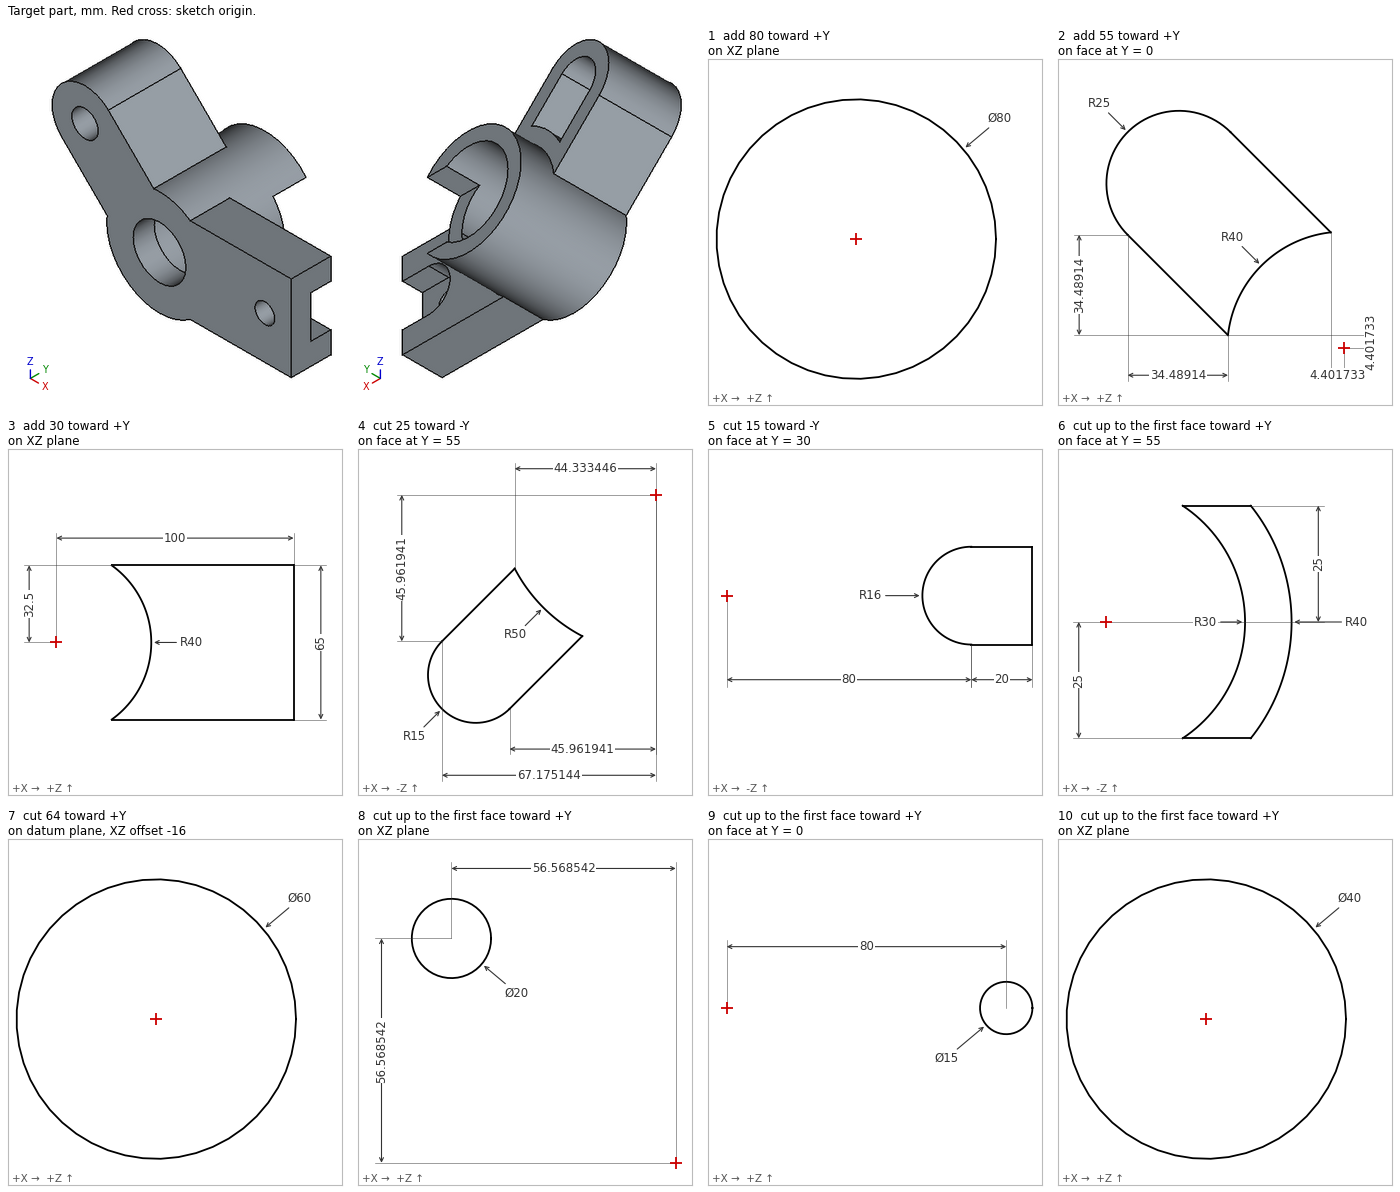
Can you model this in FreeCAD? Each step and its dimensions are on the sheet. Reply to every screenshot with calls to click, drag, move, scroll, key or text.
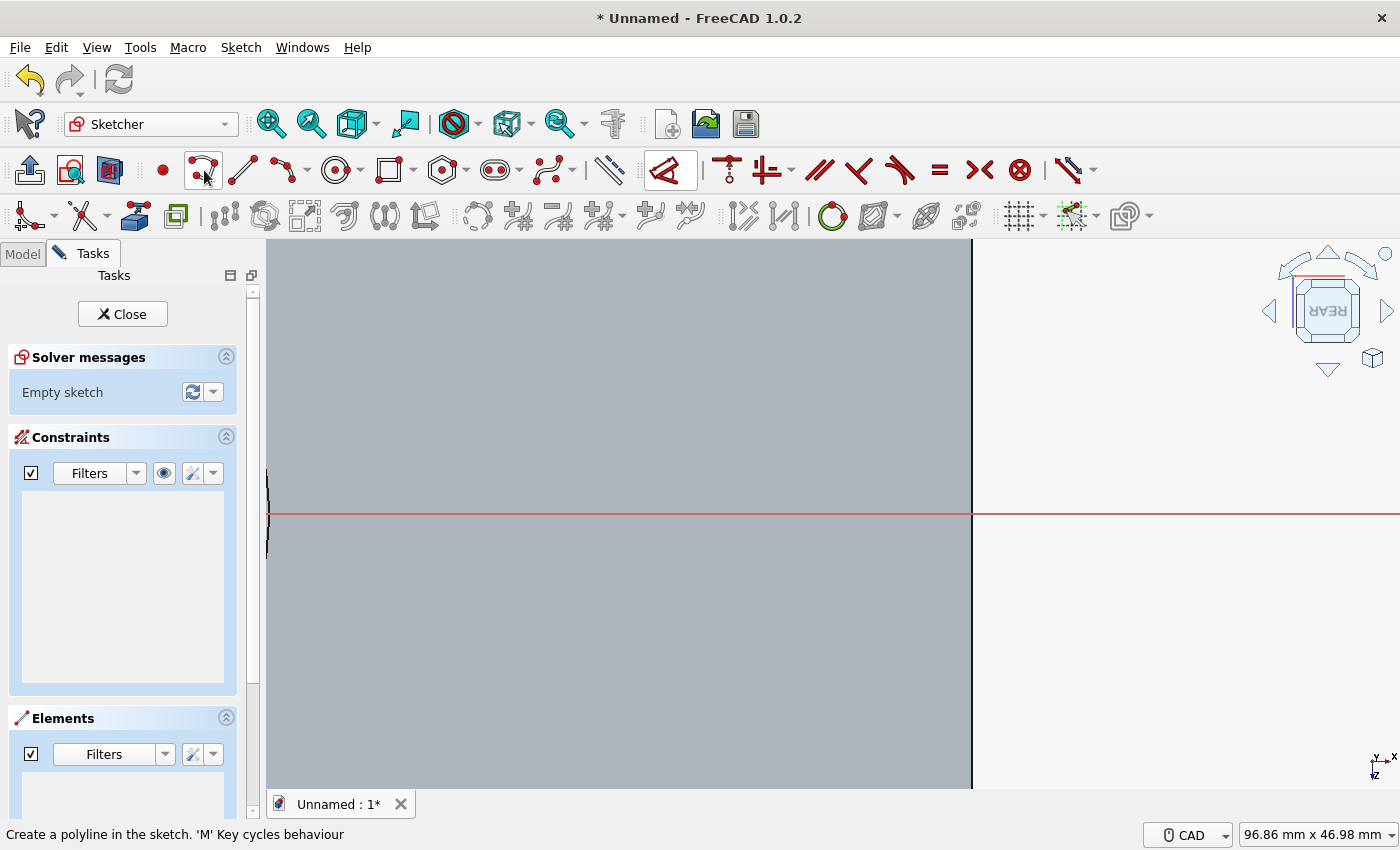
click(738, 702)
click(972, 702)
click(972, 327)
click(738, 327)
right_click(738, 327)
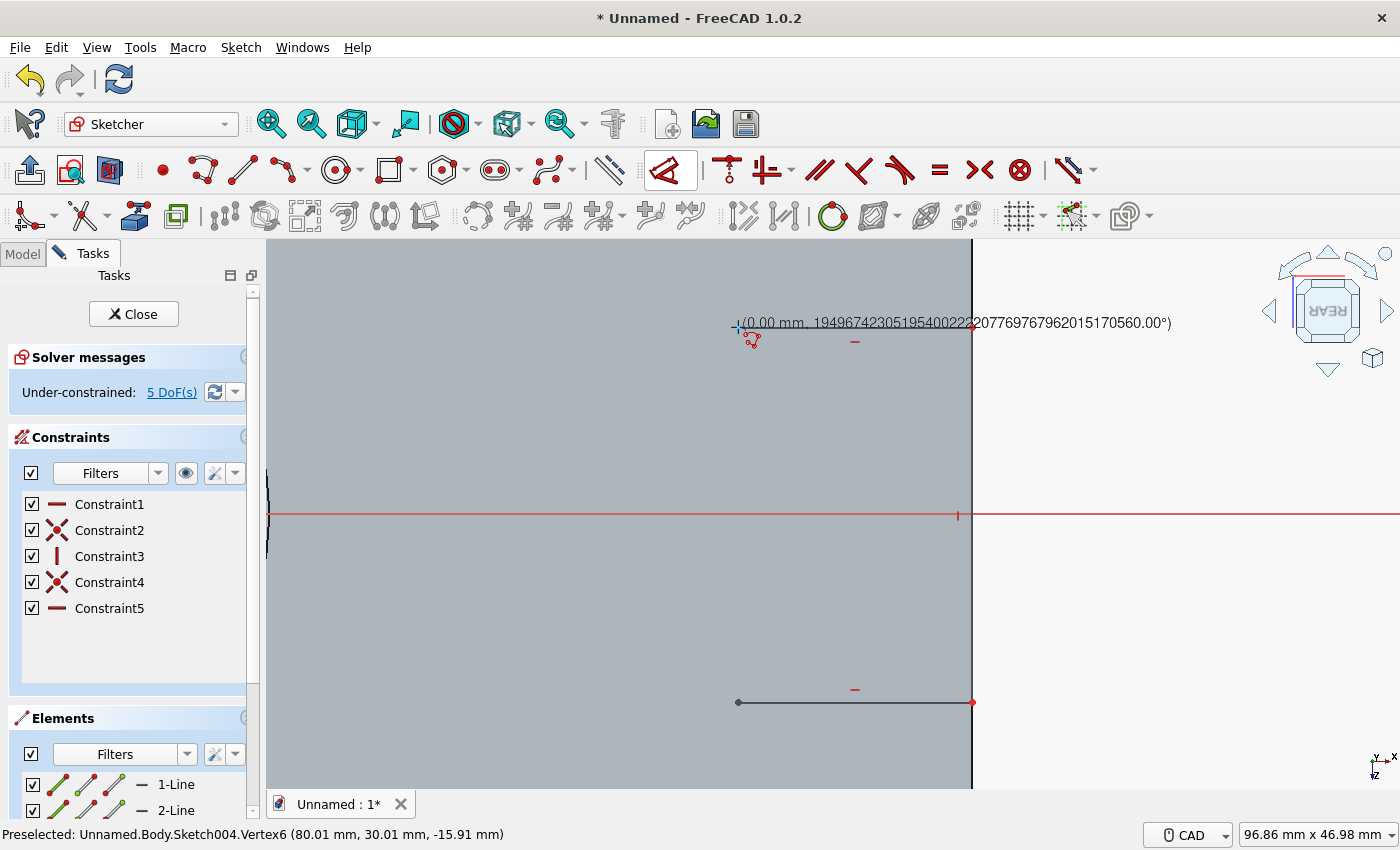
click(284, 170)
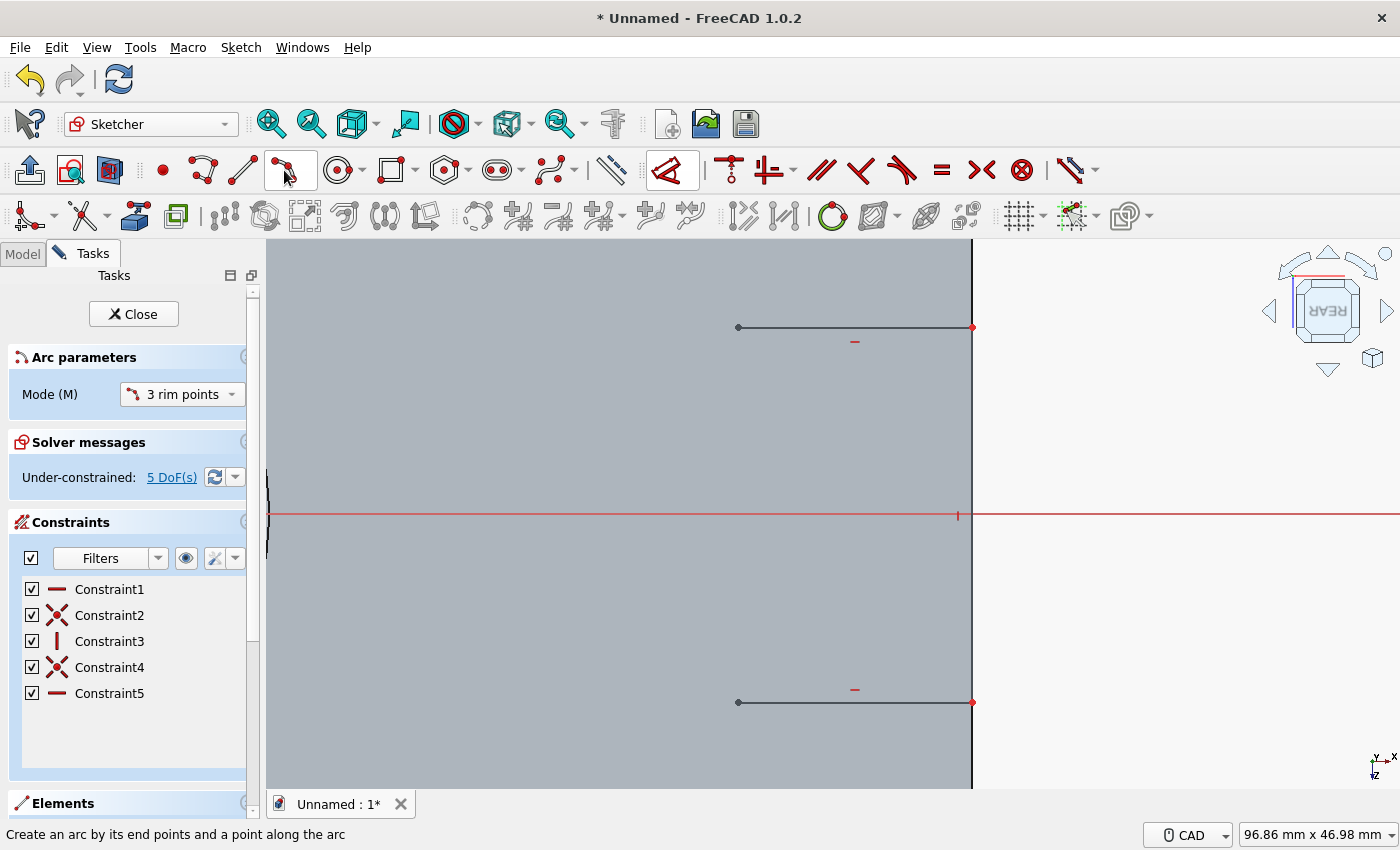
click(738, 328)
click(738, 703)
click(560, 456)
key(Escape)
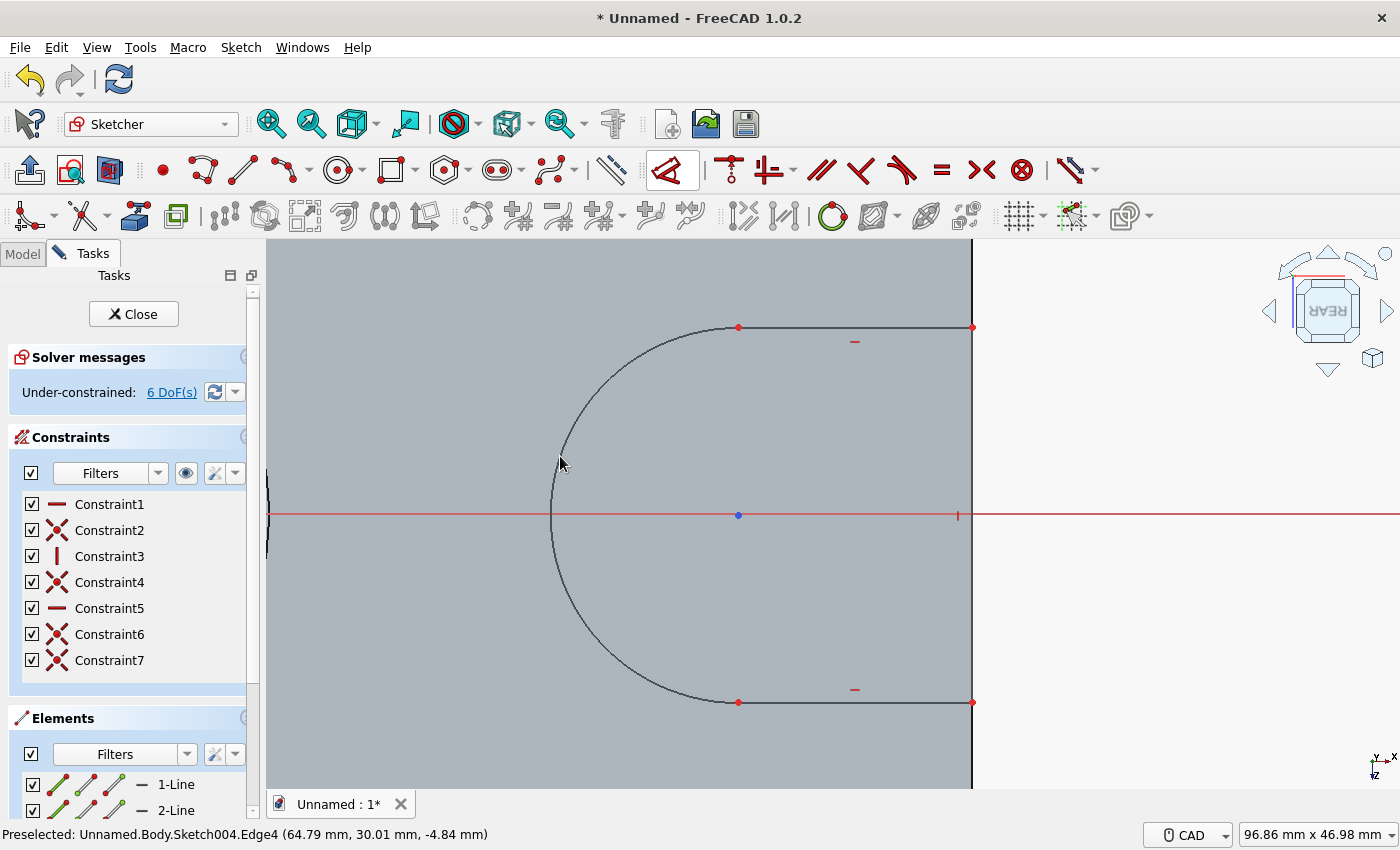
click(808, 703)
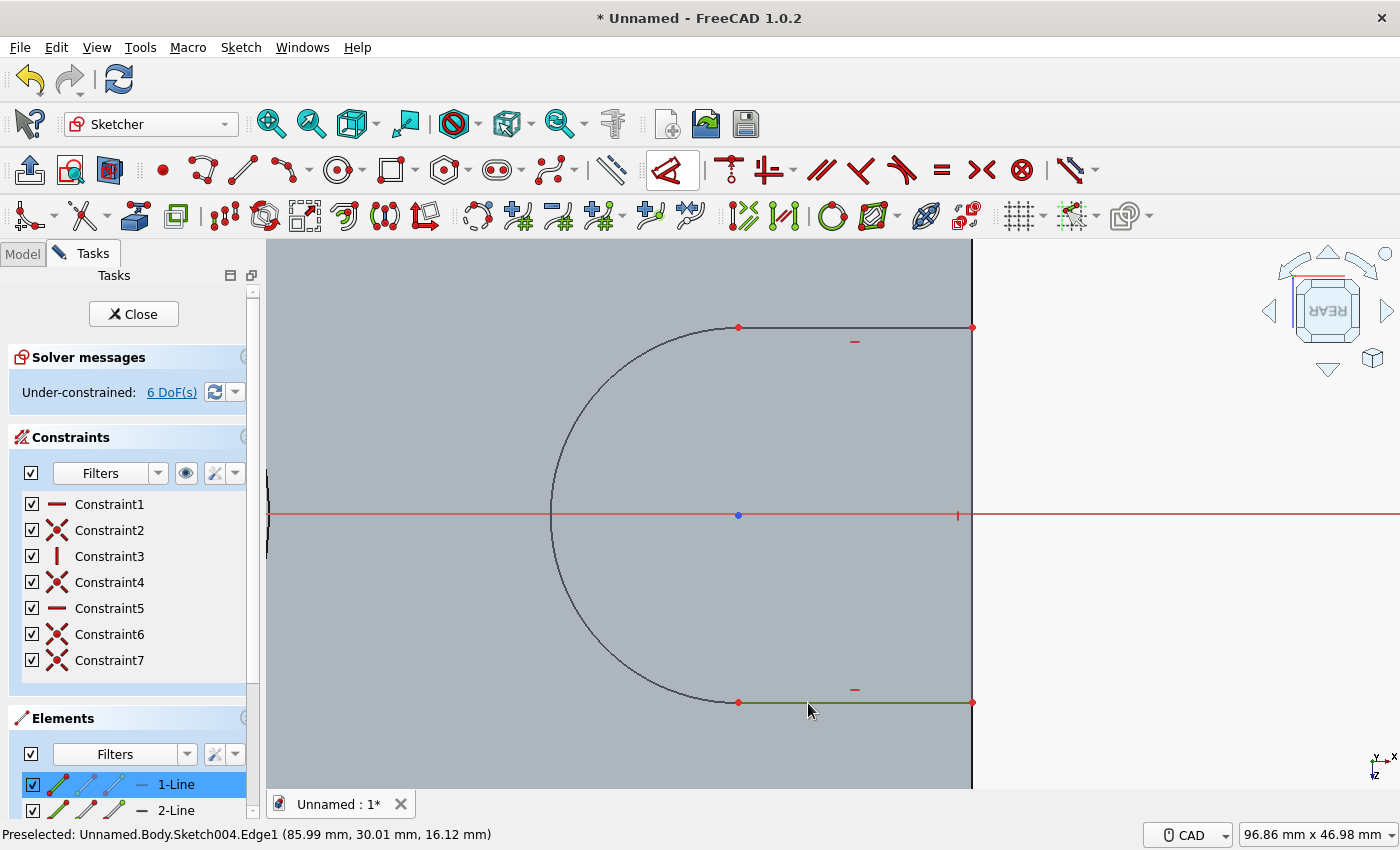
click(586, 405)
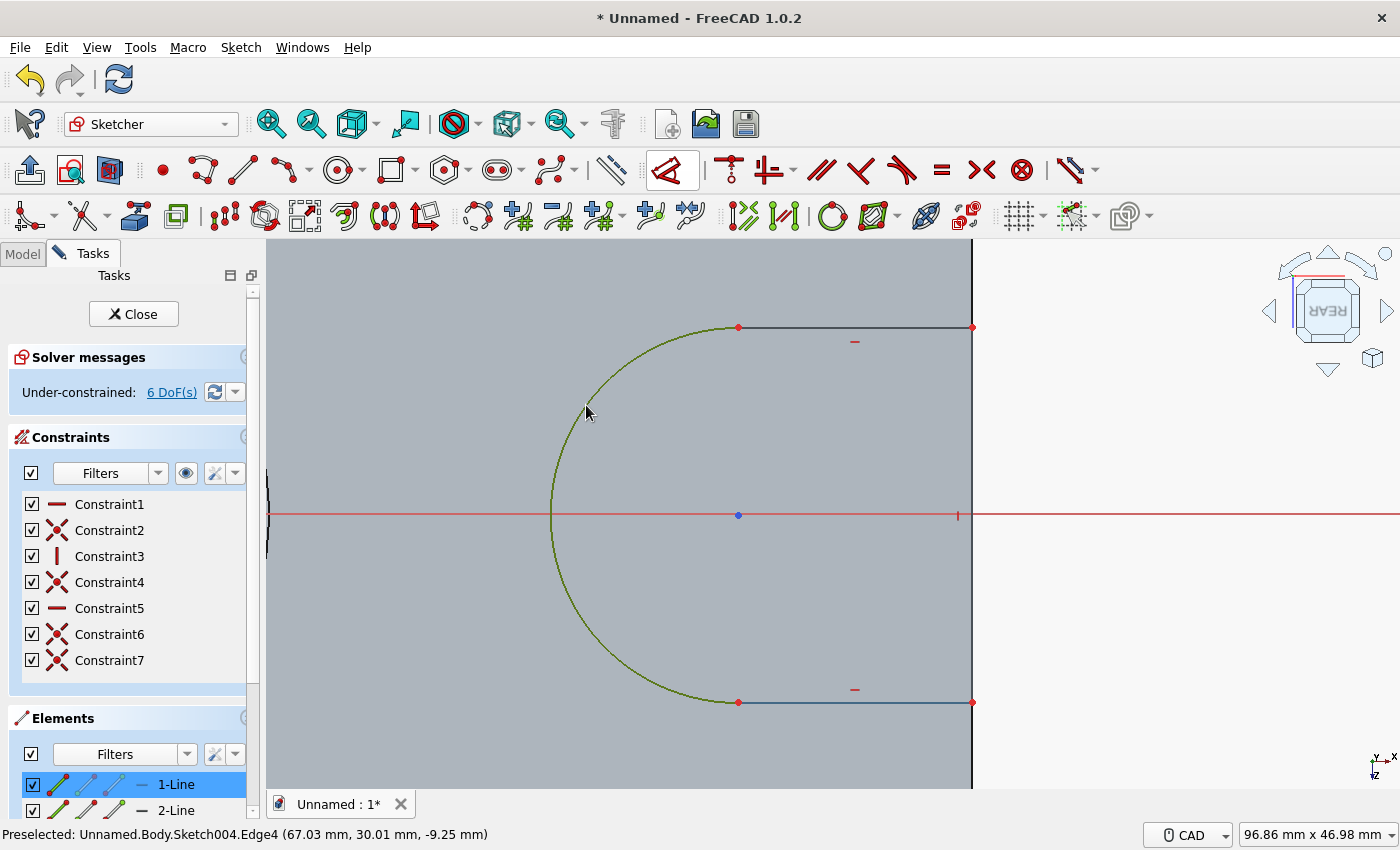
click(902, 170)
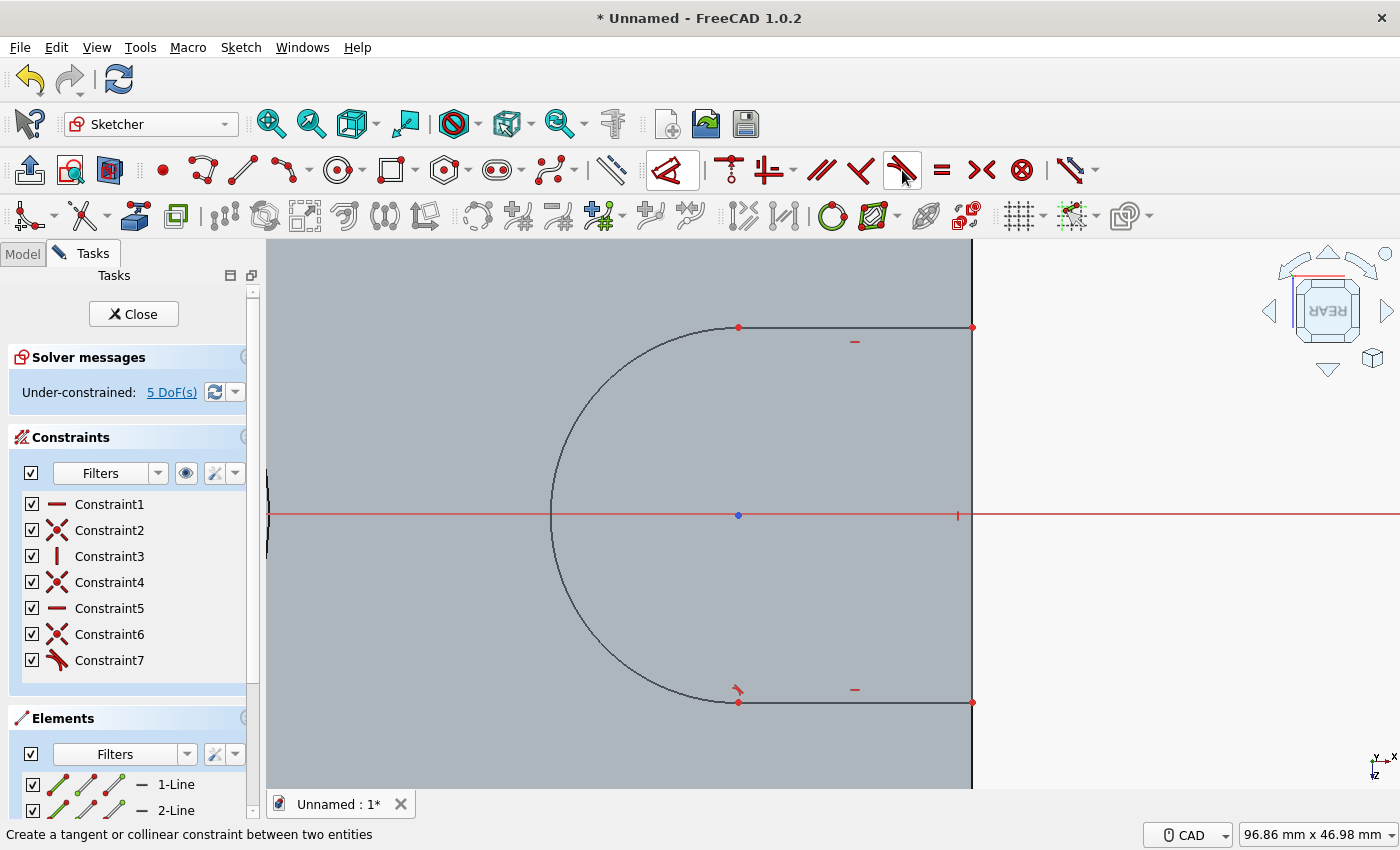
click(902, 328)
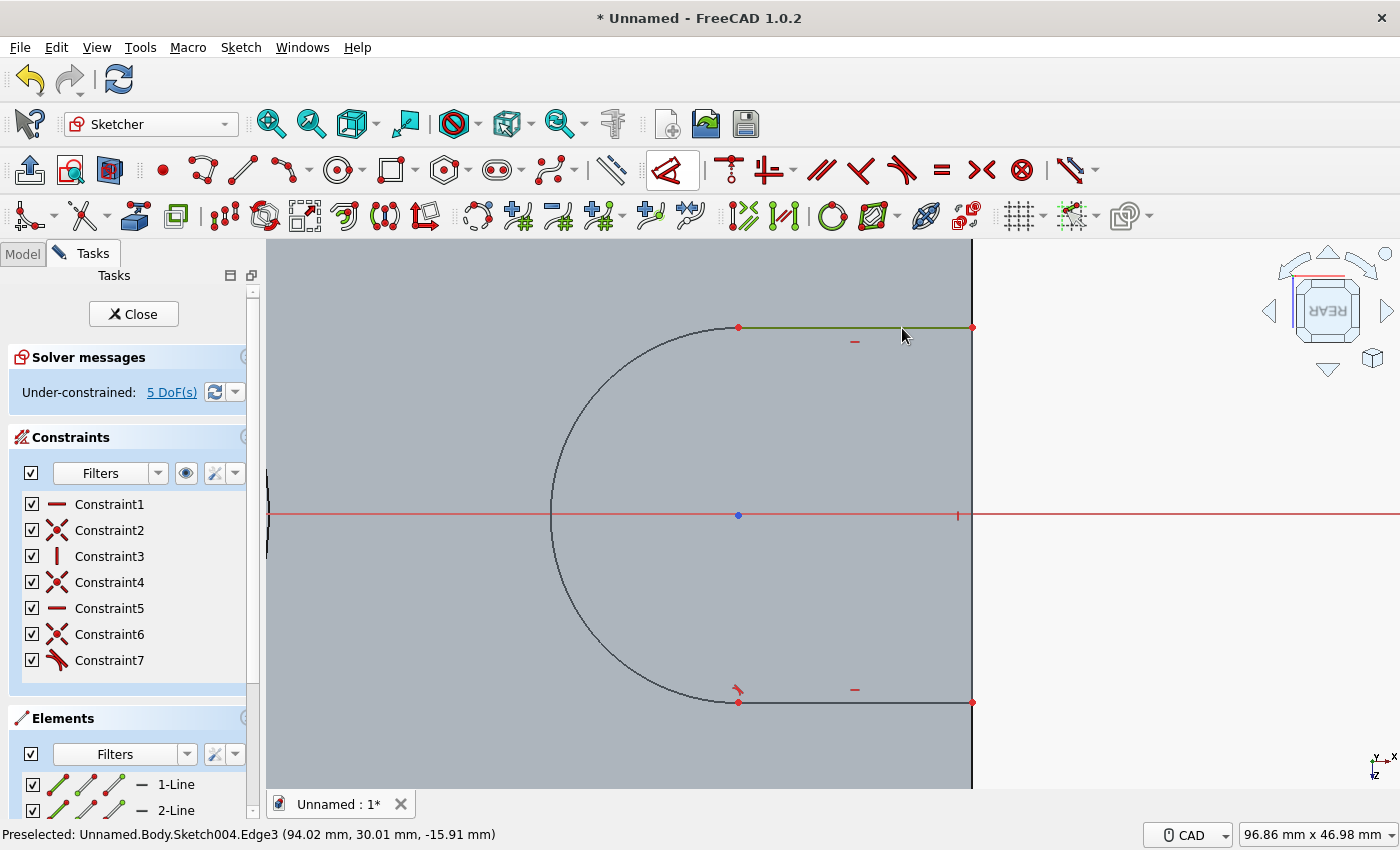
click(586, 405)